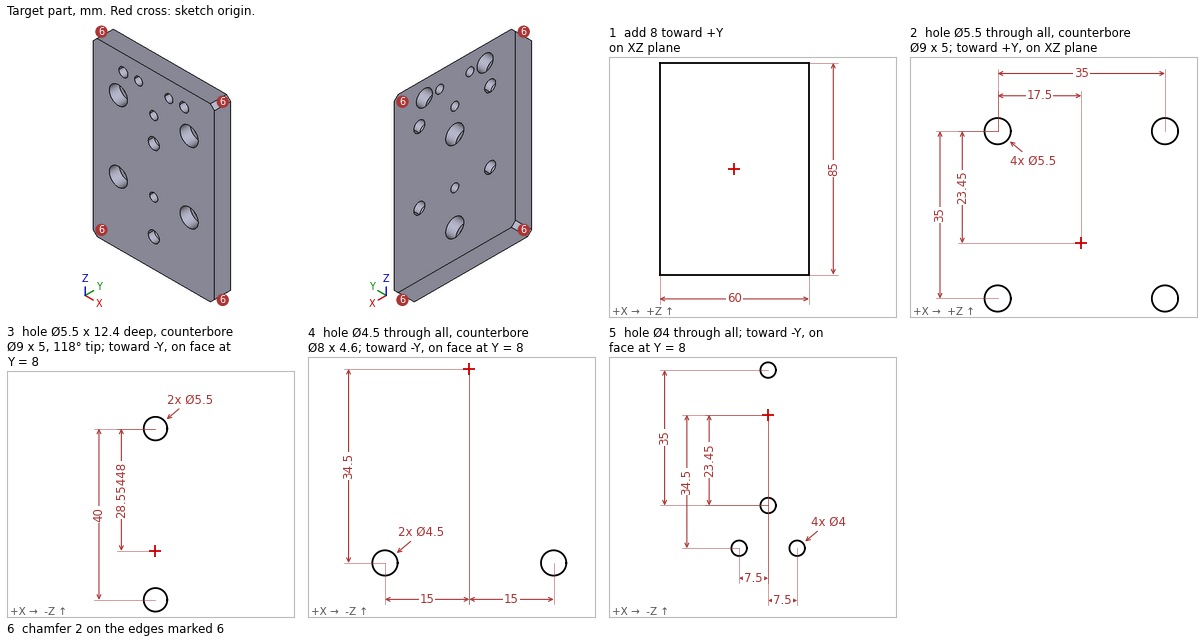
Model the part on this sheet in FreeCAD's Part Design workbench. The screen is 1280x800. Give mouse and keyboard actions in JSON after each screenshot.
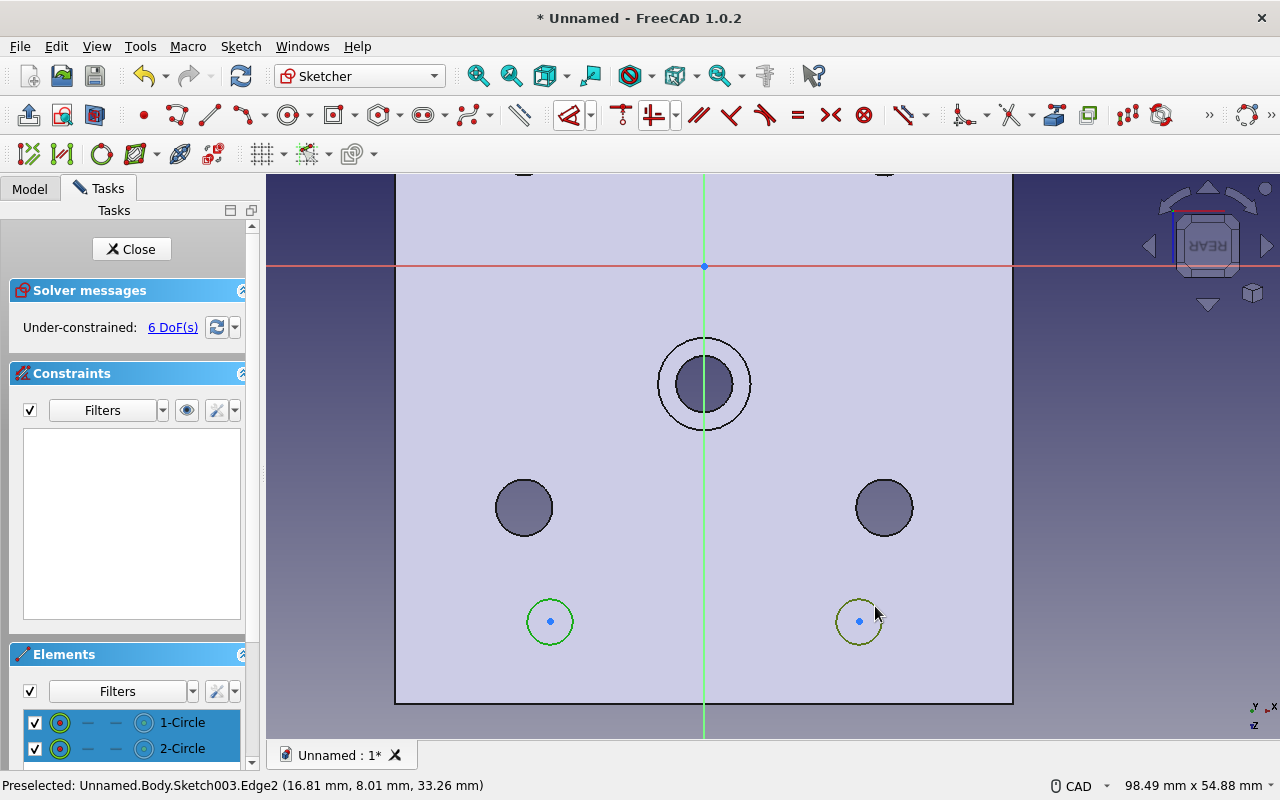
{"action": "left_click", "coordinate": [798, 116]}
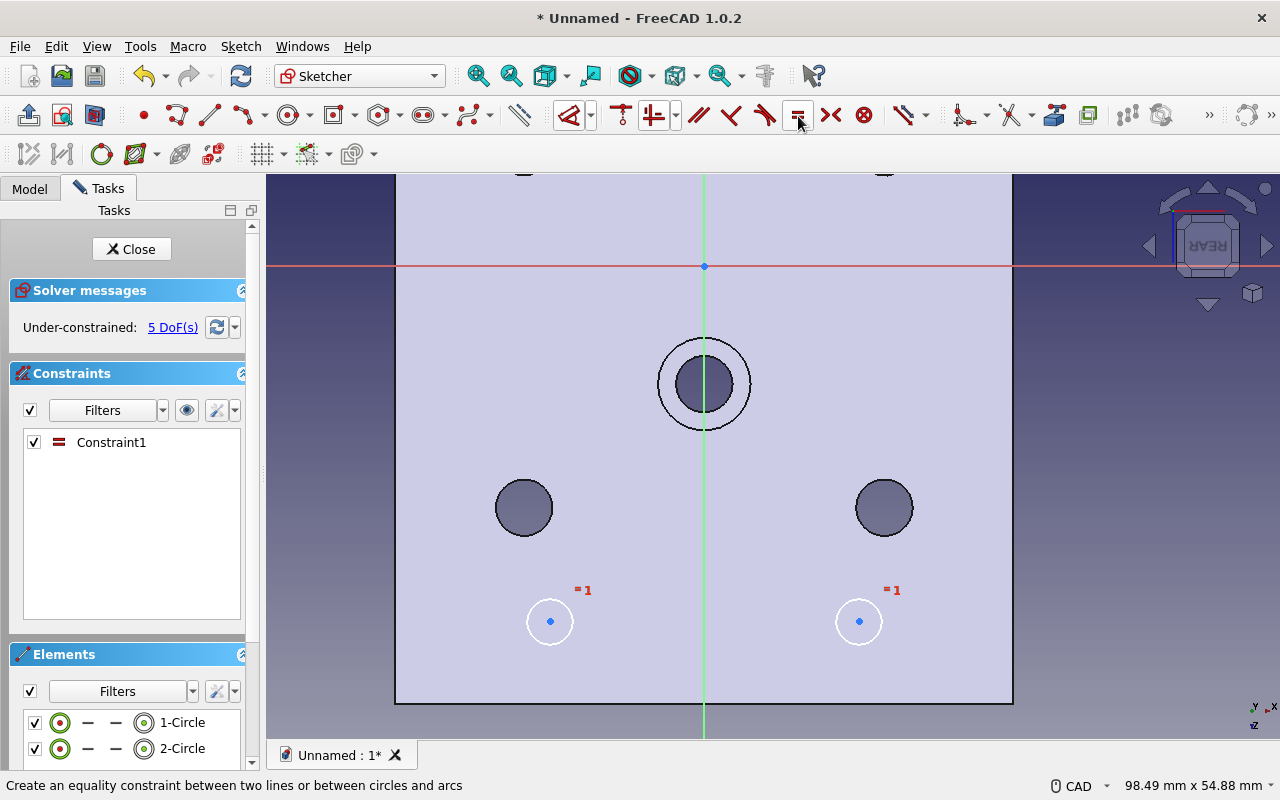
{"action": "left_click", "coordinate": [550, 622]}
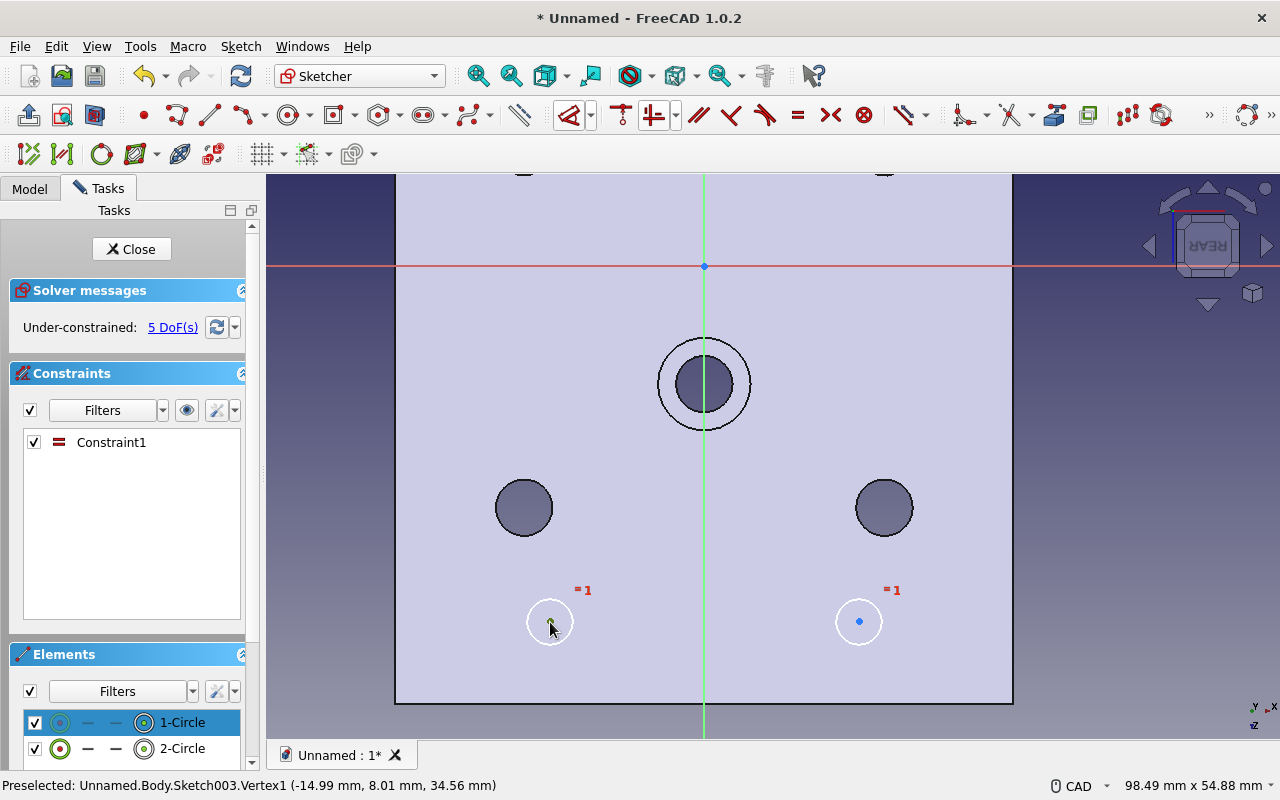
{"action": "left_click", "coordinate": [859, 622]}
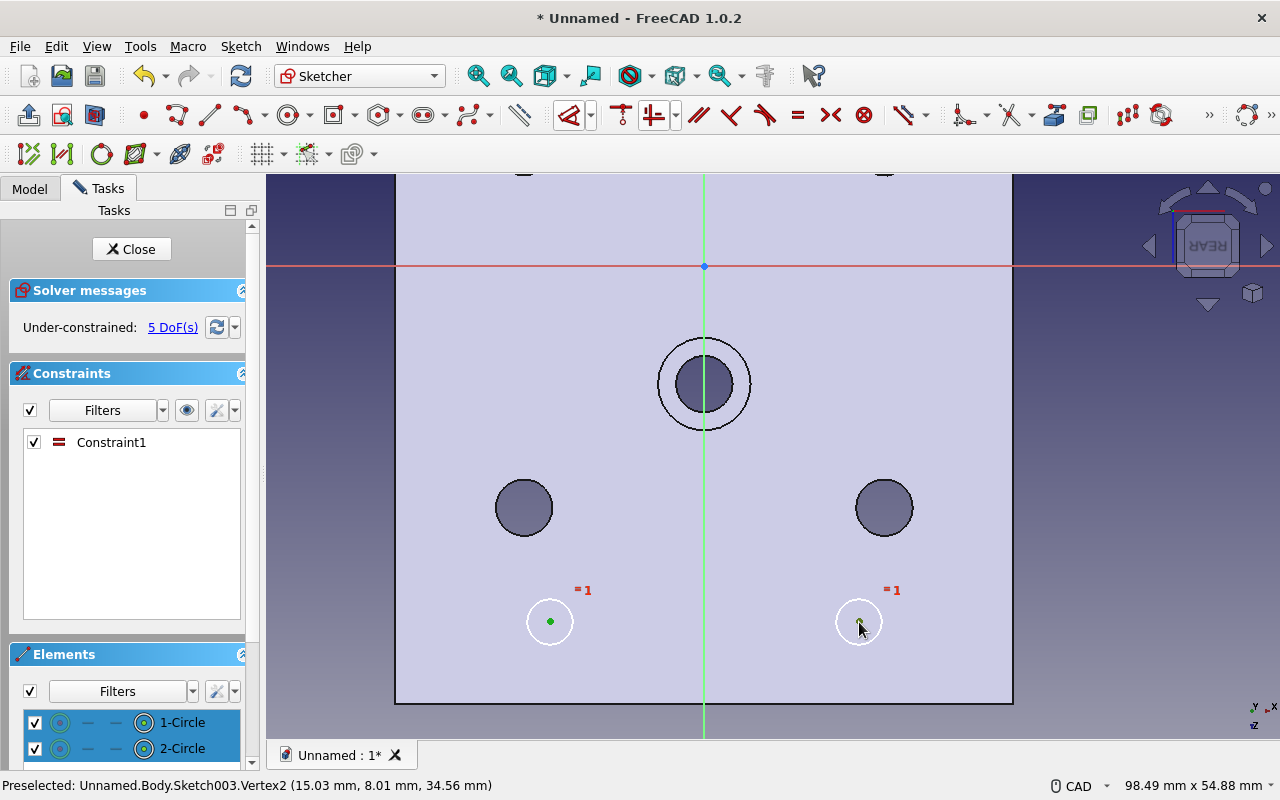
{"action": "left_click", "coordinate": [676, 116]}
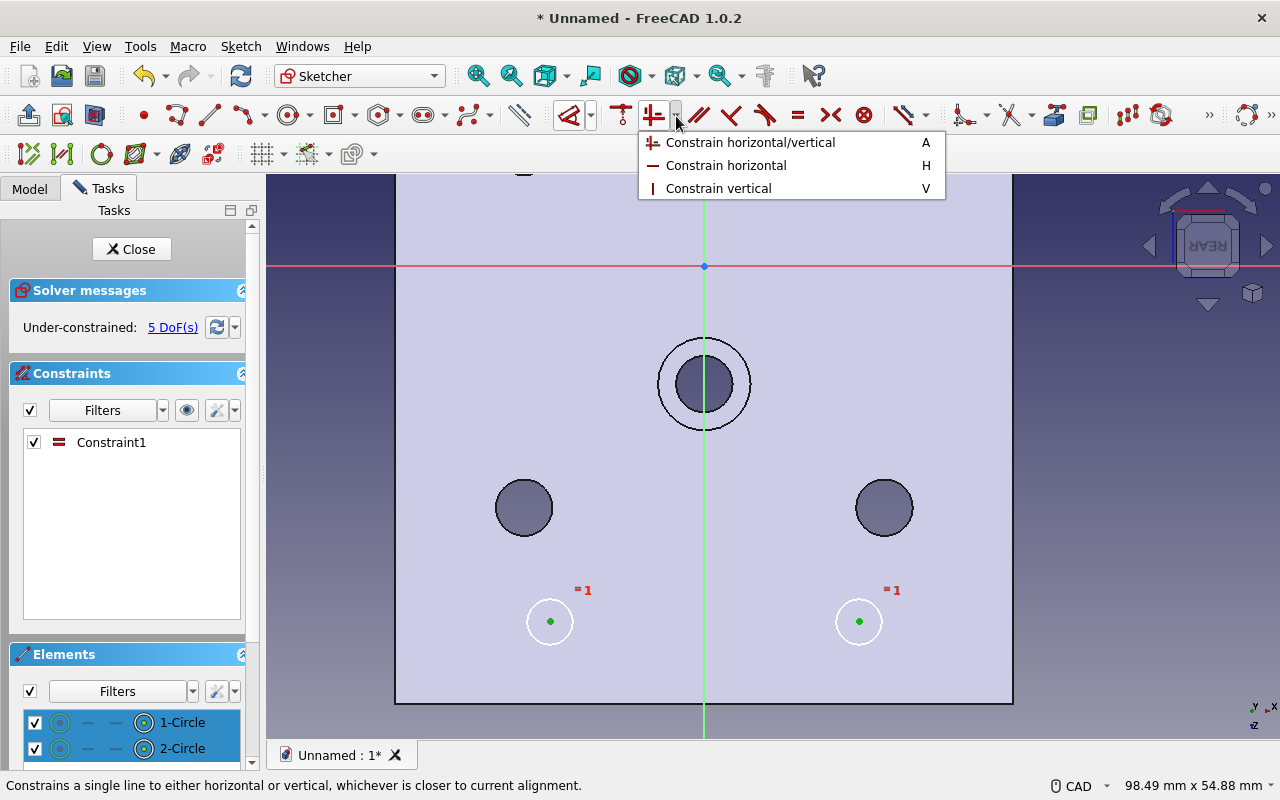
{"action": "left_click", "coordinate": [792, 166]}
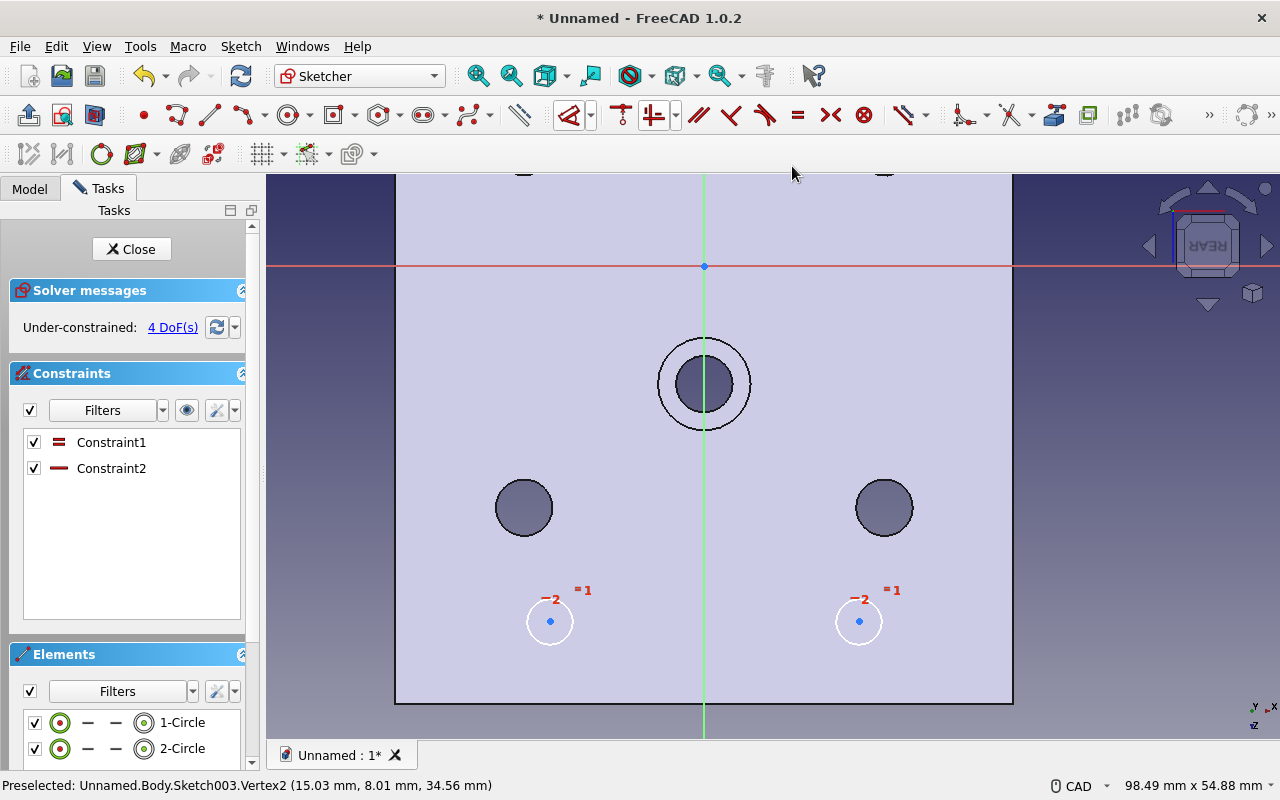
{"action": "left_click", "coordinate": [566, 606]}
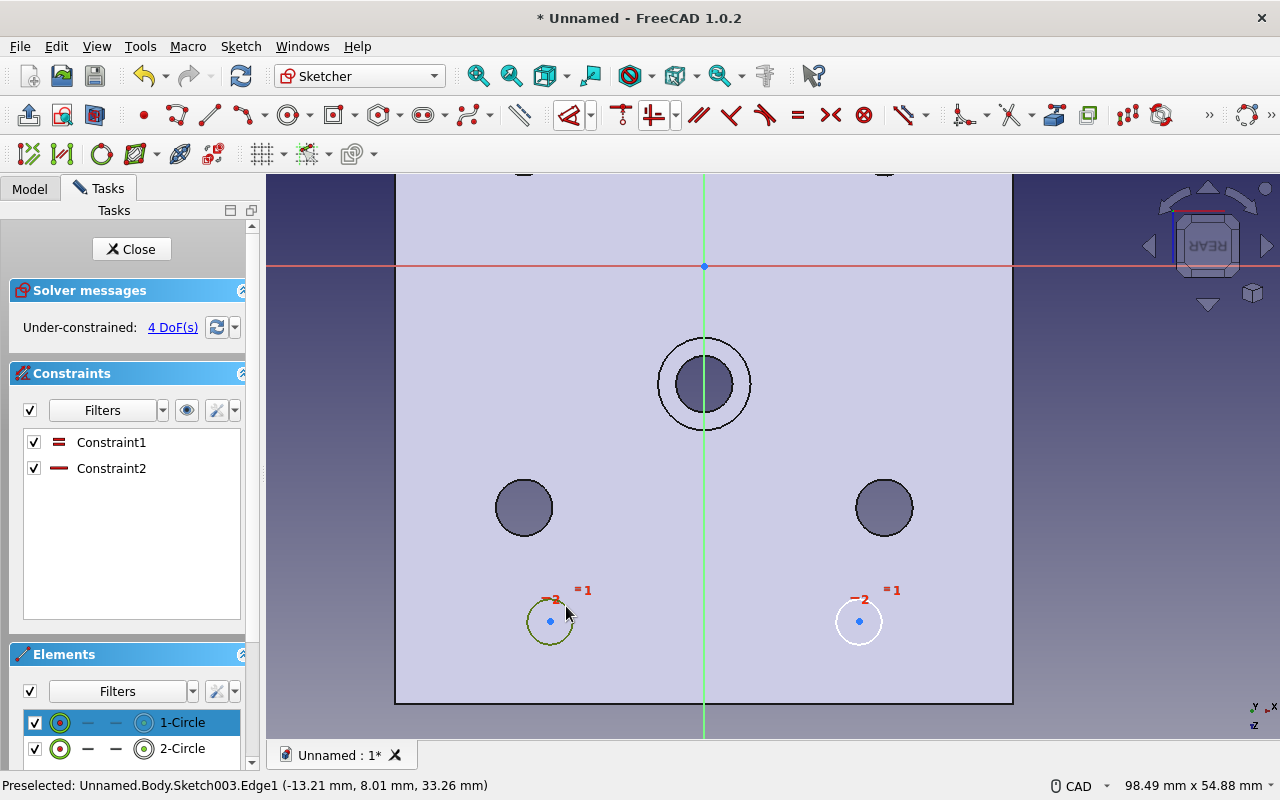
{"action": "key", "text": "k o"}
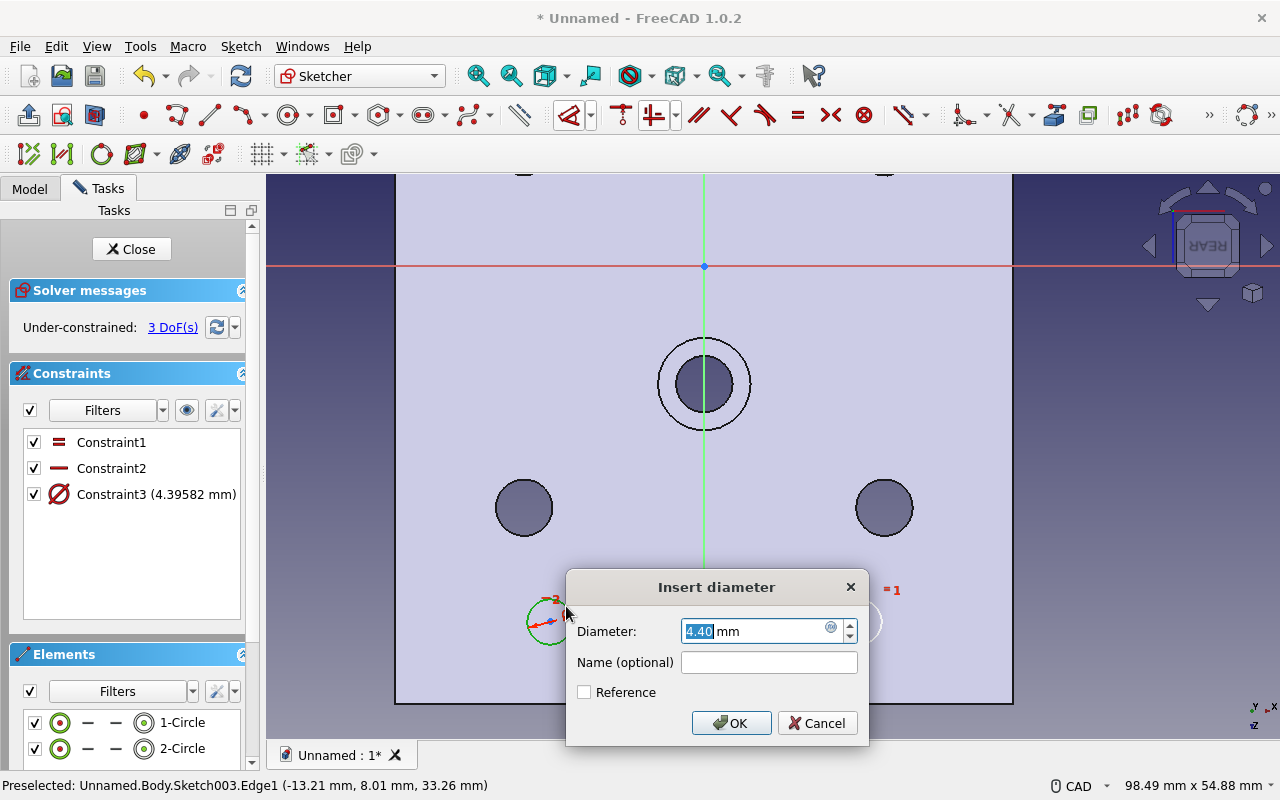
{"action": "type", "text": "4.5"}
{"action": "key", "text": "Return"}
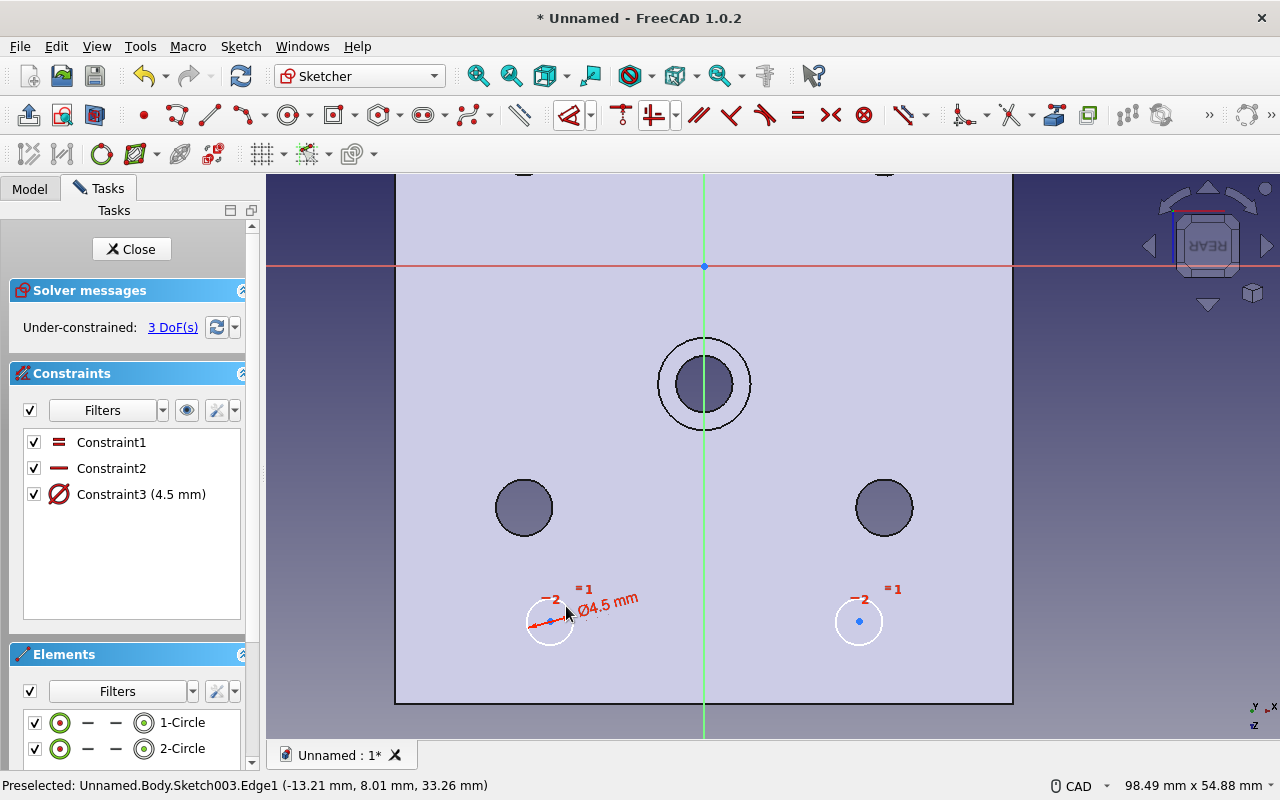
{"action": "left_click", "coordinate": [550, 622]}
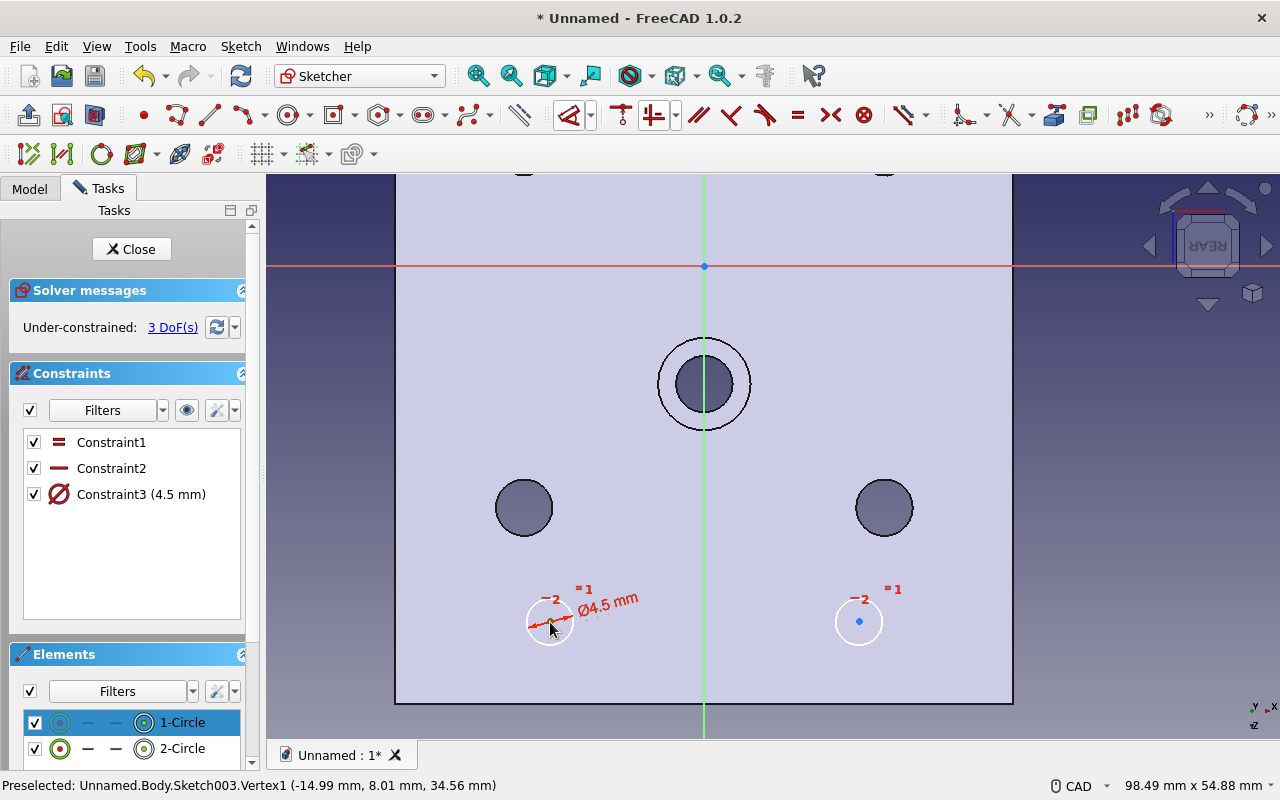
{"action": "key", "text": "l"}